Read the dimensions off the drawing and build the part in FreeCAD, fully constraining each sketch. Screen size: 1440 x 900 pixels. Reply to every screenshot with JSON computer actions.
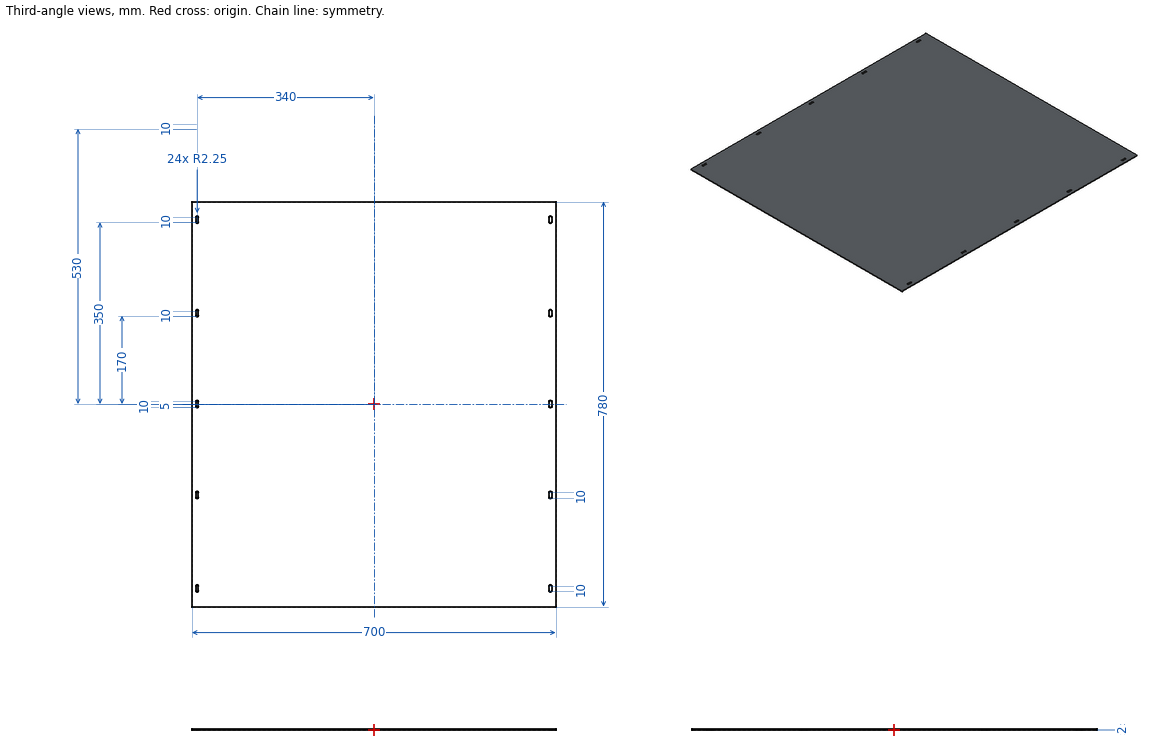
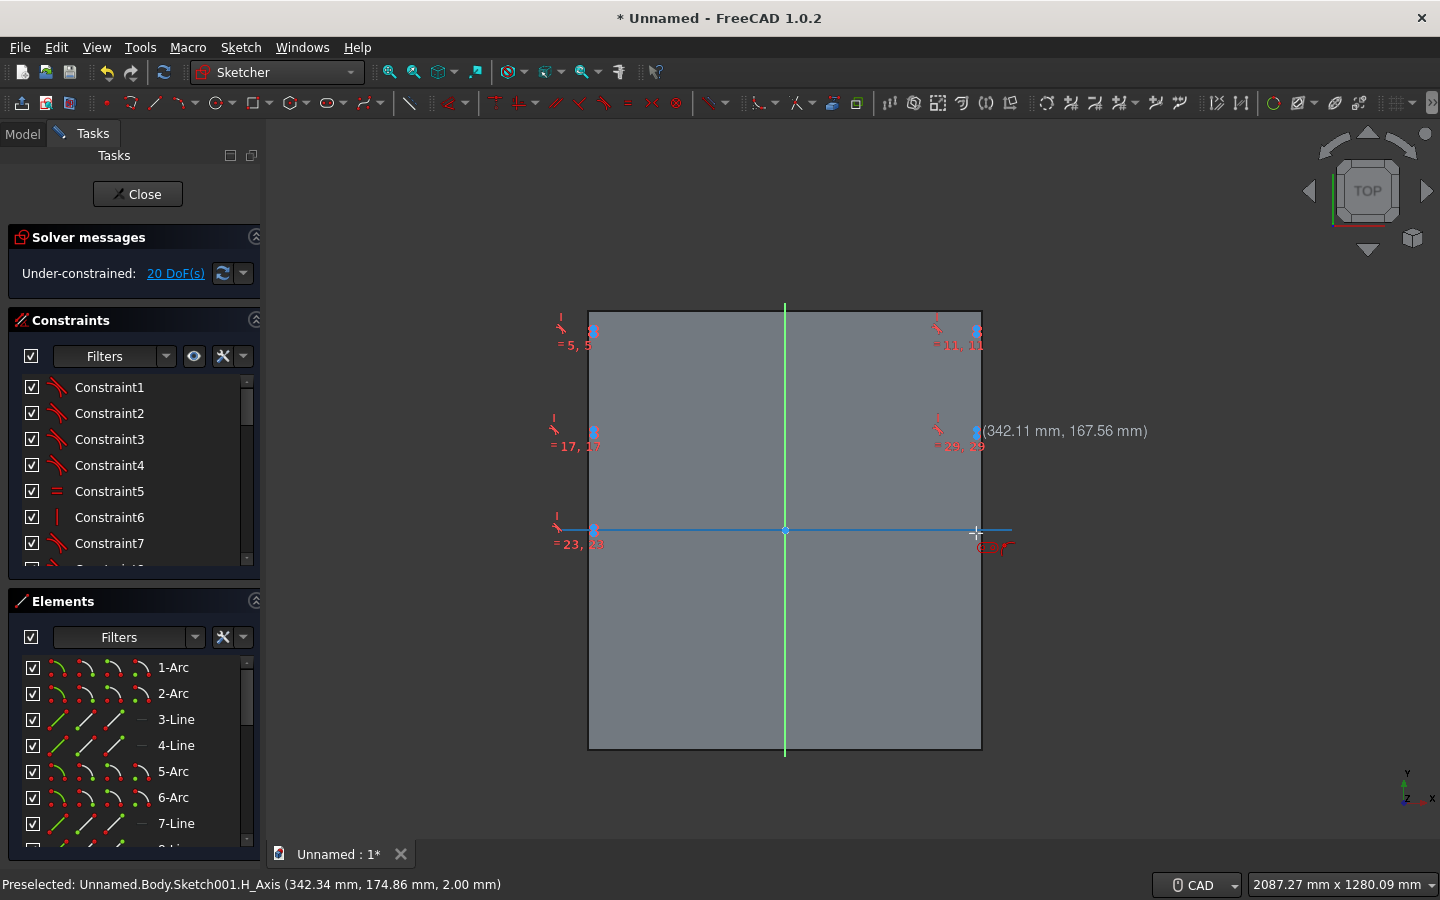
{"action": "scroll", "coordinate": [976, 533], "scroll_direction": "up", "scroll_amount": 9}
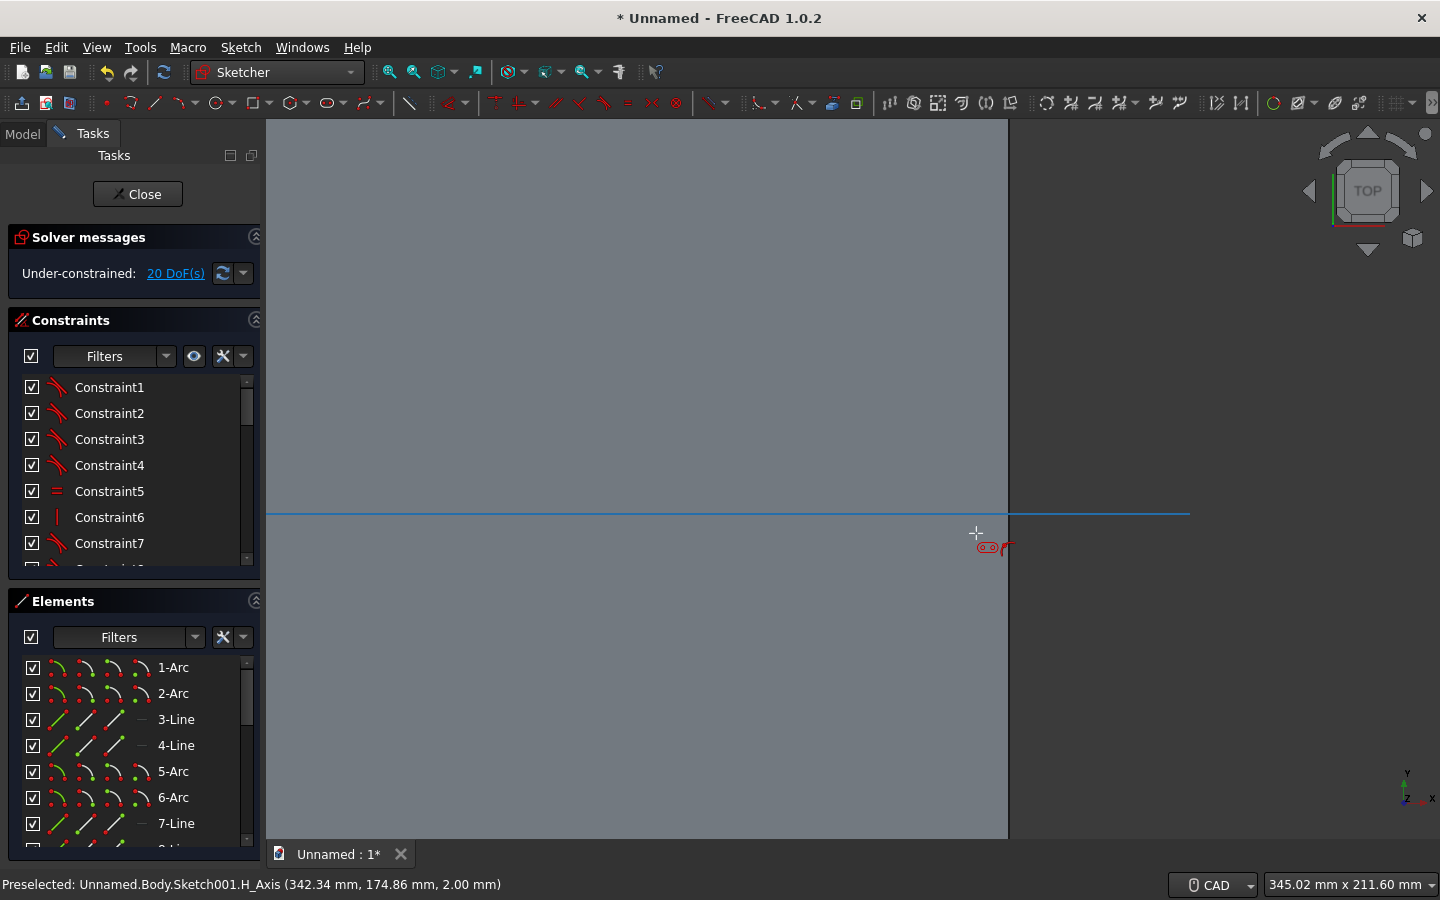
{"action": "left_click", "coordinate": [975, 531]}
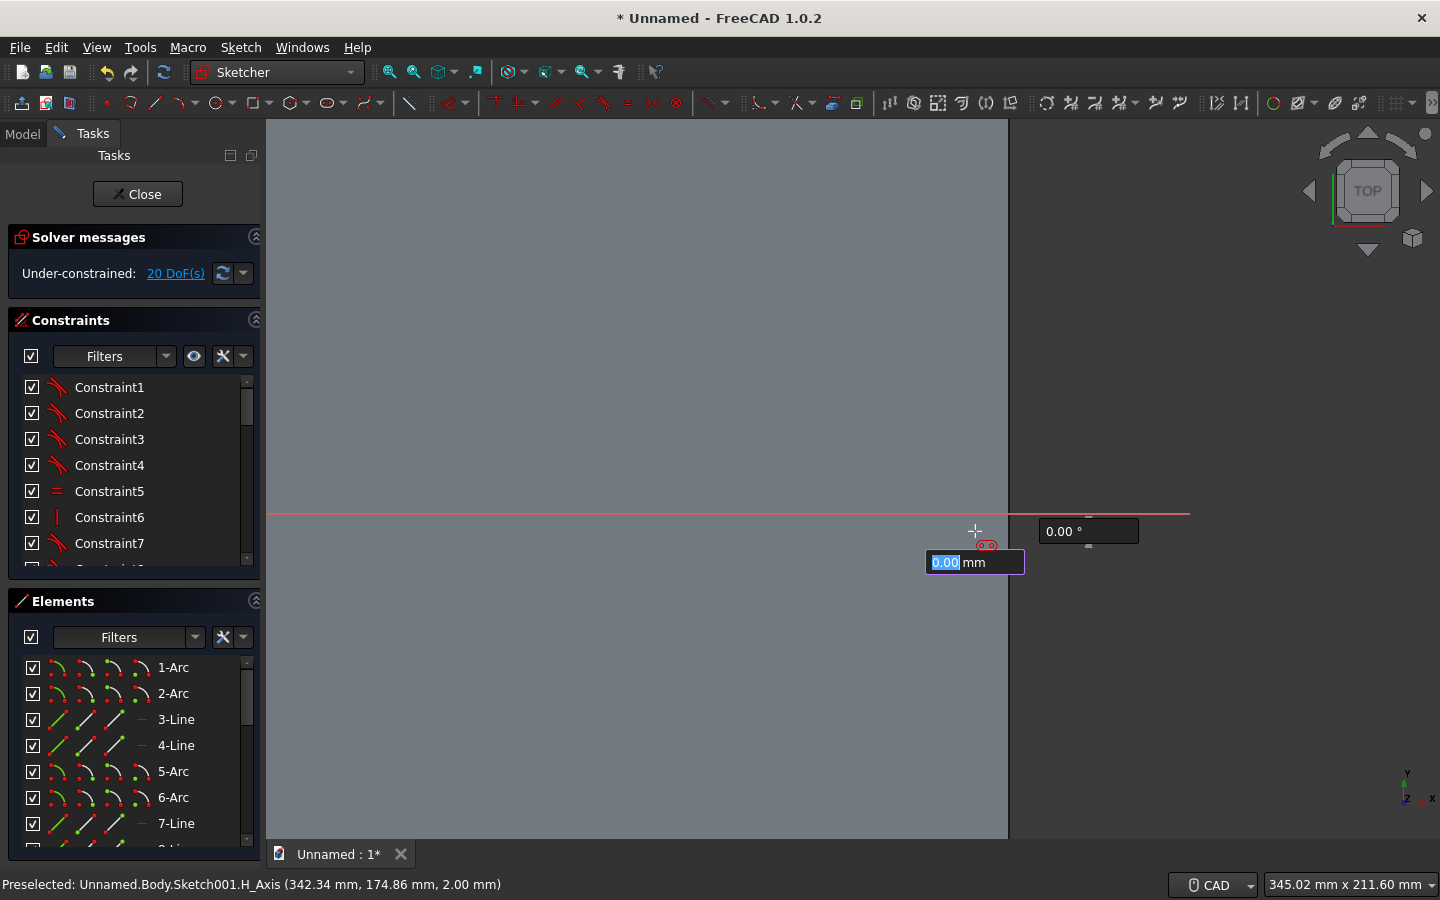
{"action": "left_click", "coordinate": [975, 497]}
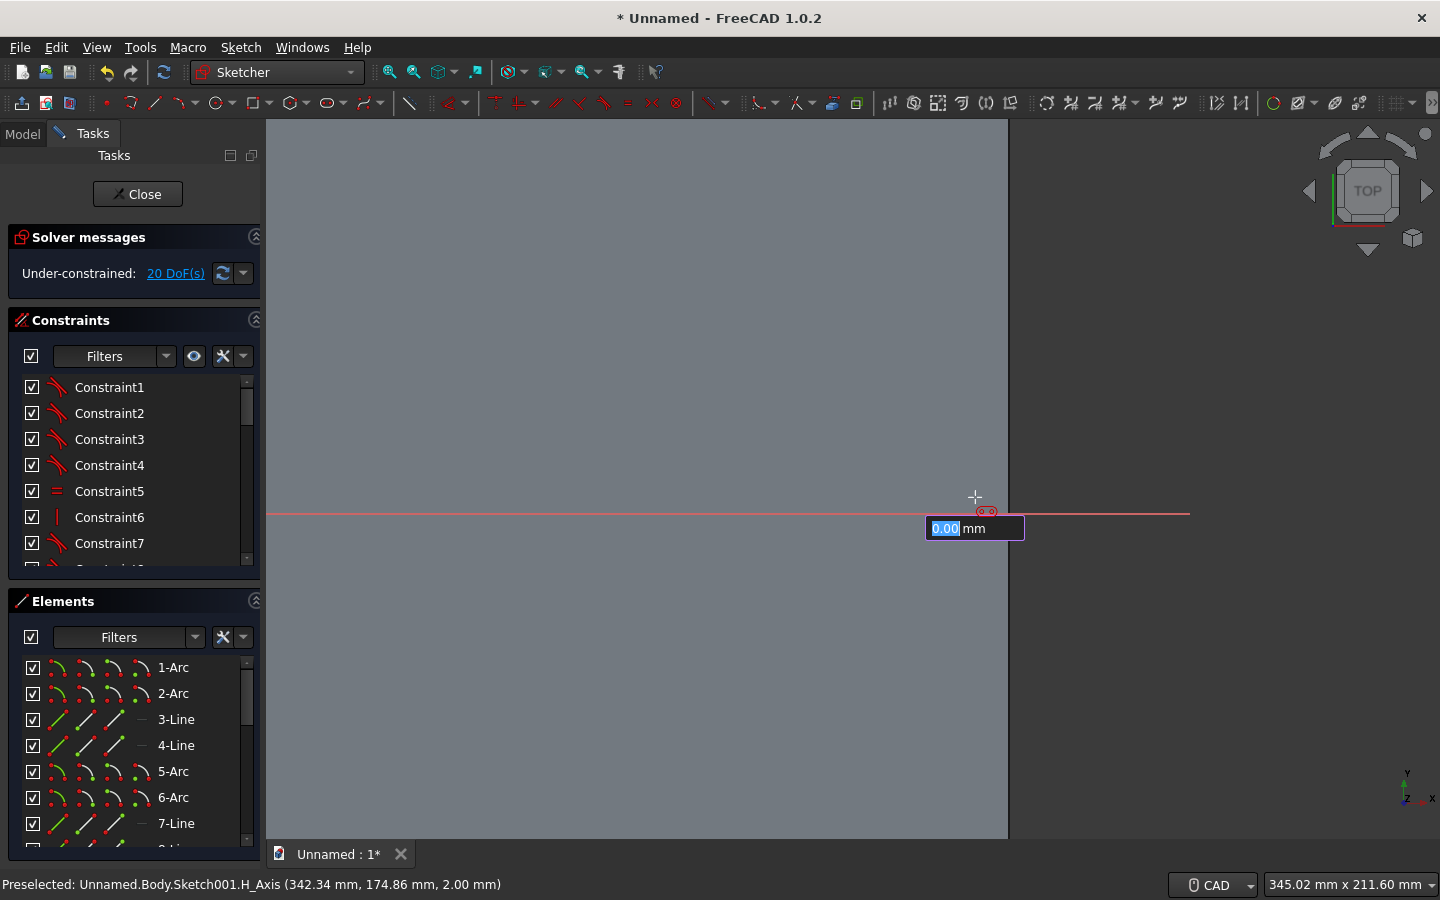
{"action": "scroll", "coordinate": [983, 519], "scroll_direction": "up", "scroll_amount": 6}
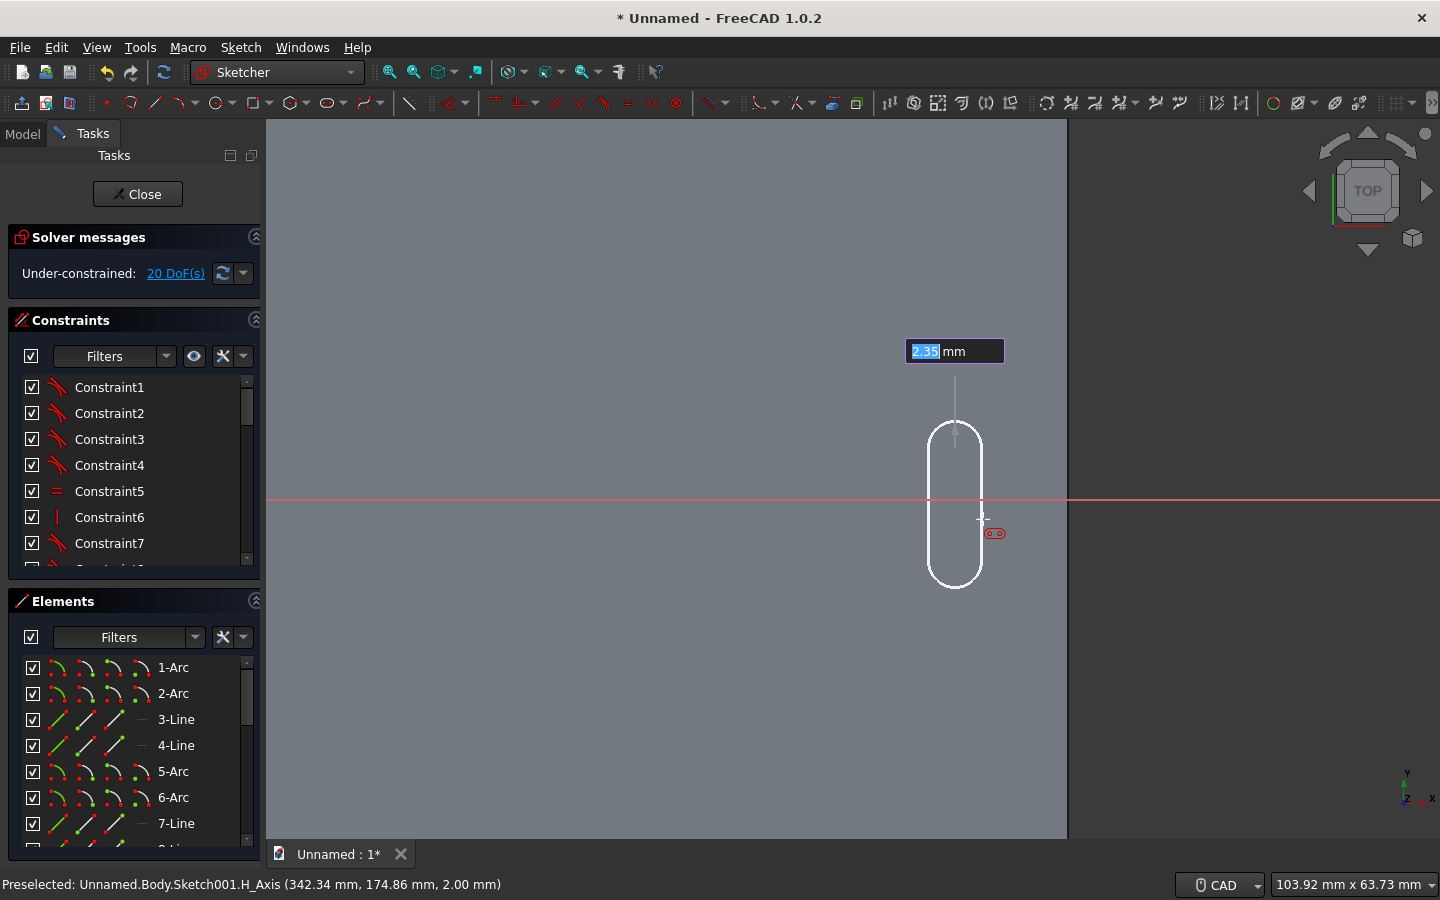
{"action": "left_click", "coordinate": [980, 517]}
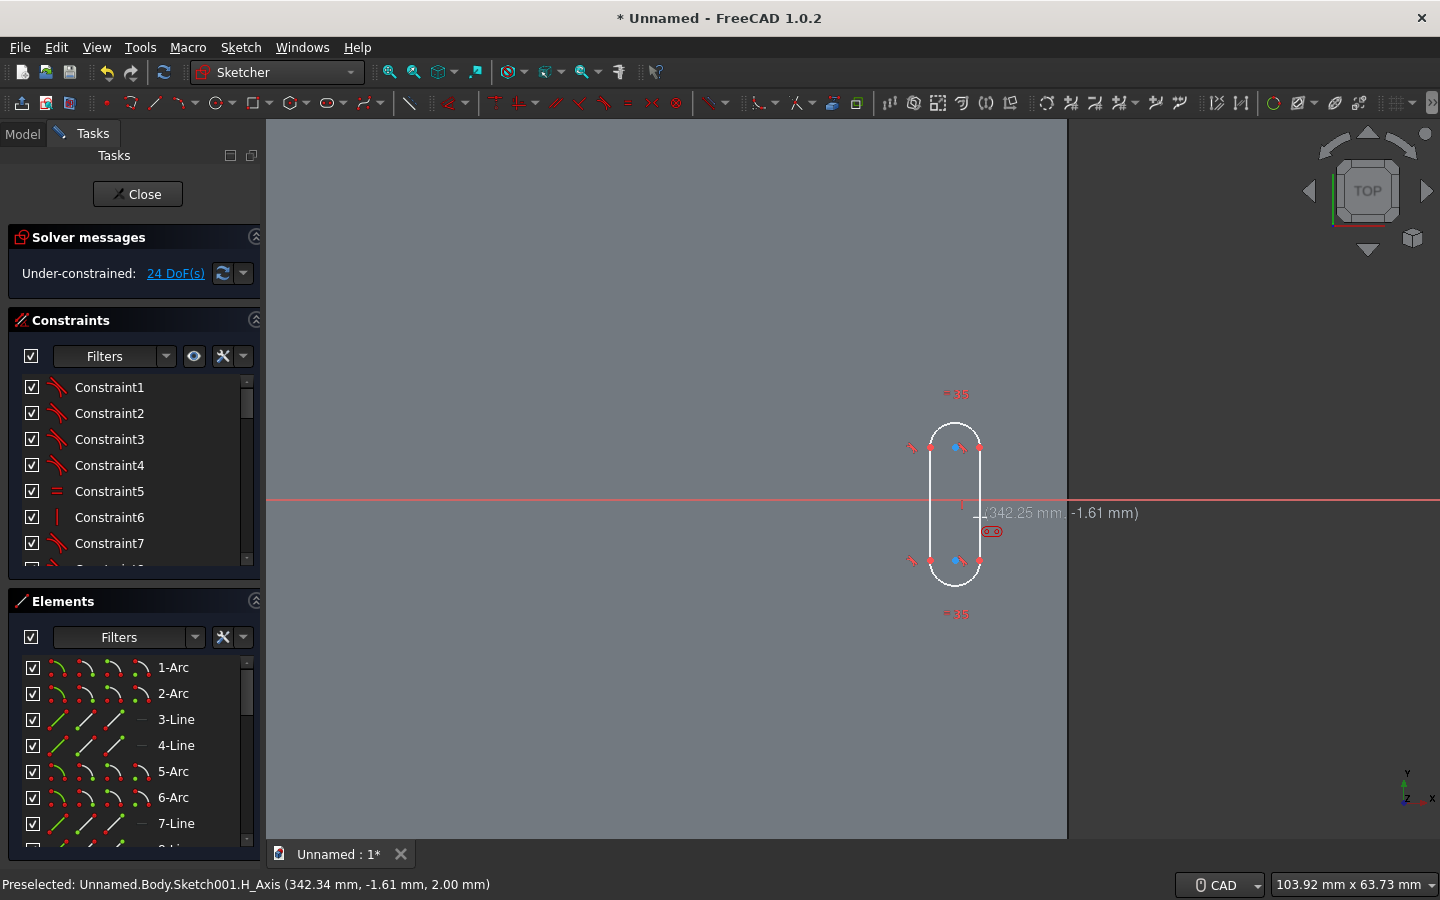
{"action": "scroll", "coordinate": [977, 531], "scroll_direction": "down", "scroll_amount": 15}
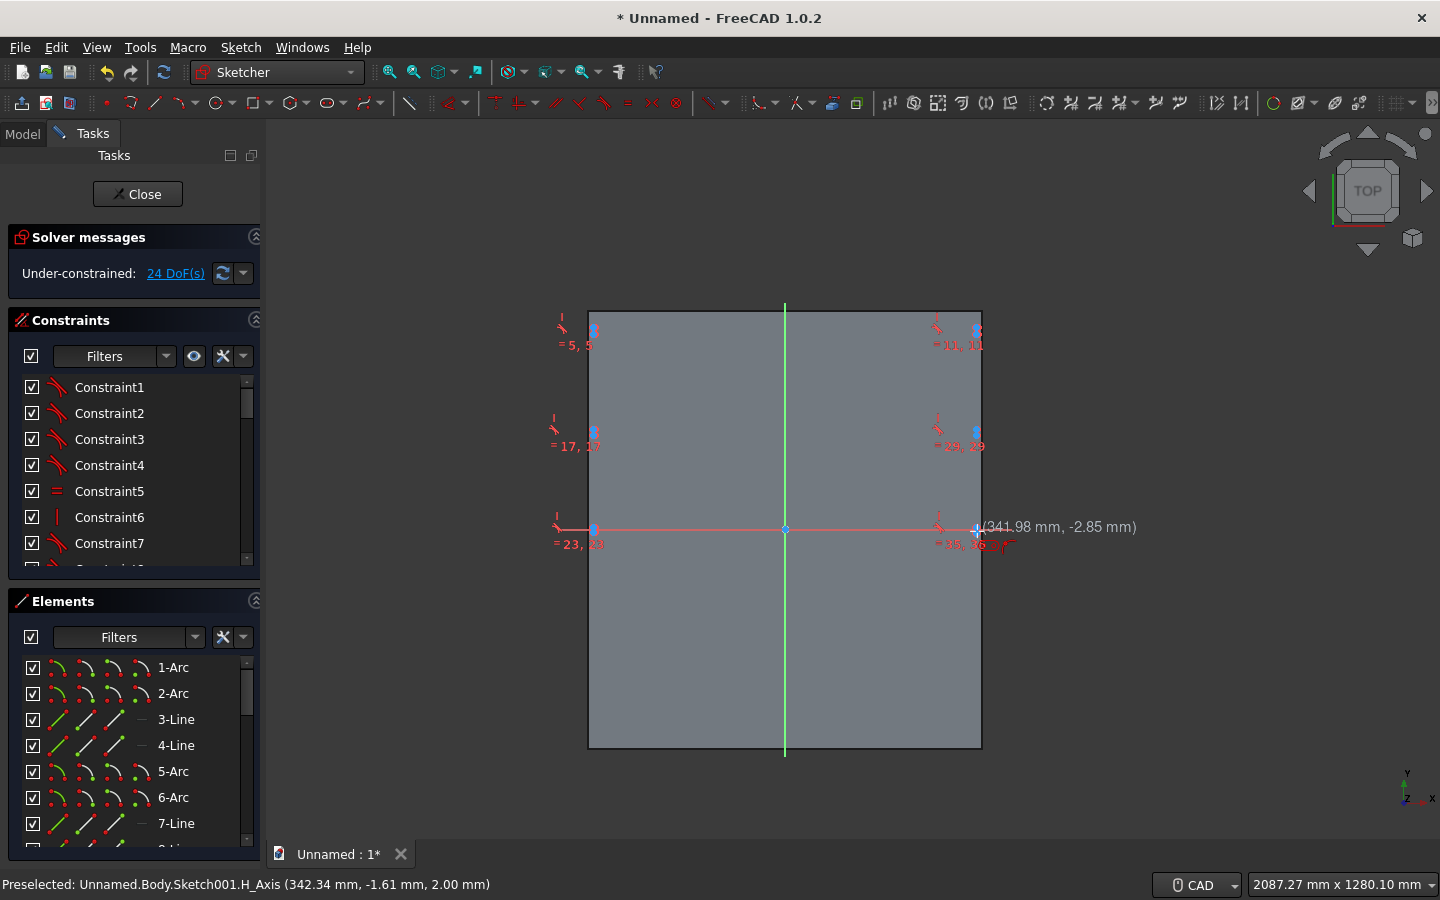
{"action": "scroll", "coordinate": [594, 232], "scroll_direction": "up", "scroll_amount": 15}